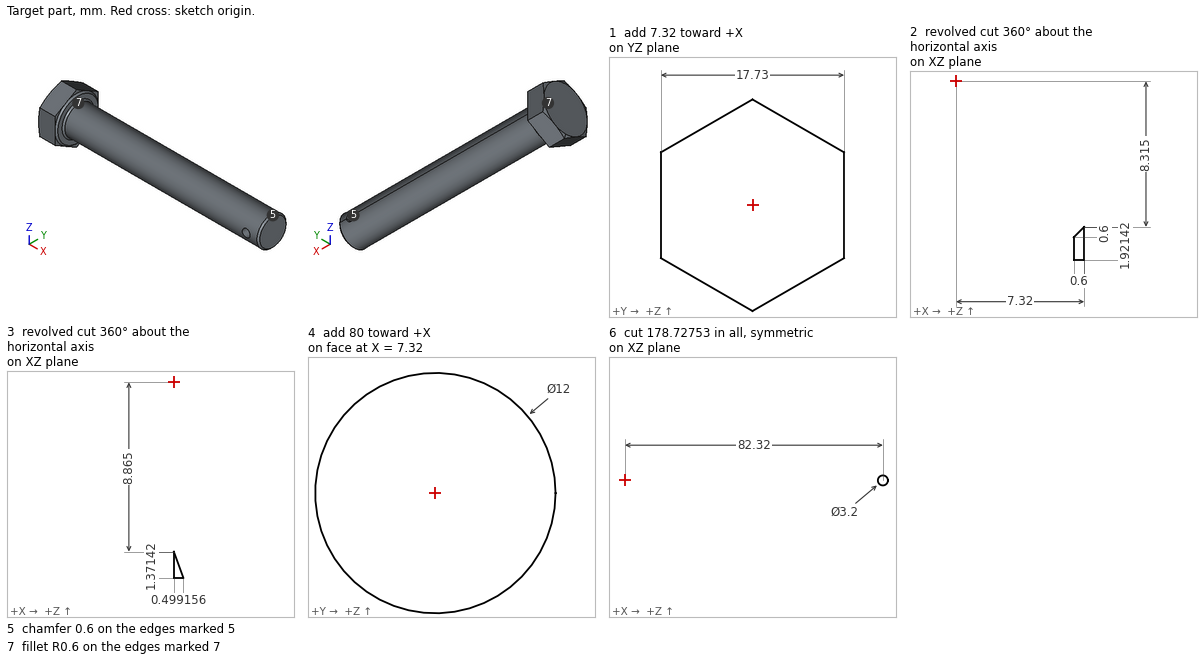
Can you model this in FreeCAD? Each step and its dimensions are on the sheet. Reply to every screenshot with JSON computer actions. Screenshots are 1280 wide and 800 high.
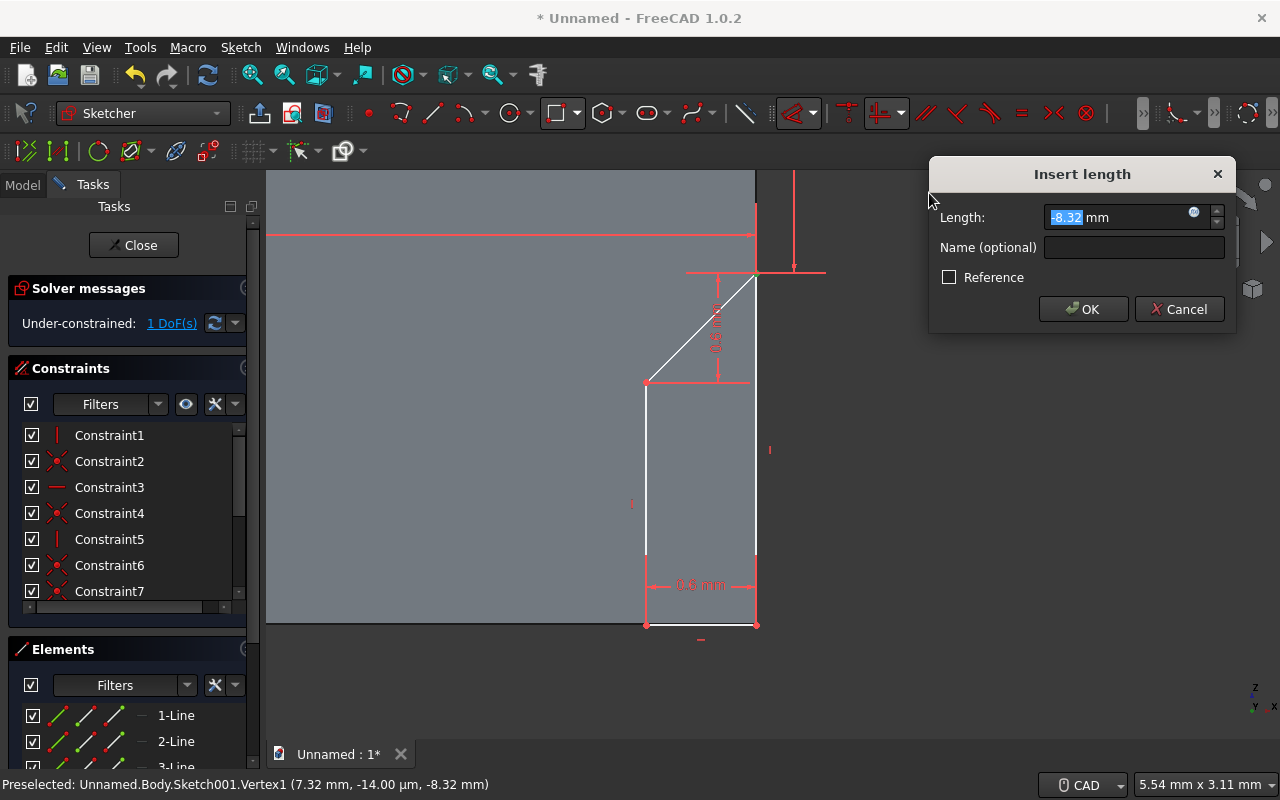
{"action": "type", "text": "-8.315"}
{"action": "key", "text": "Return"}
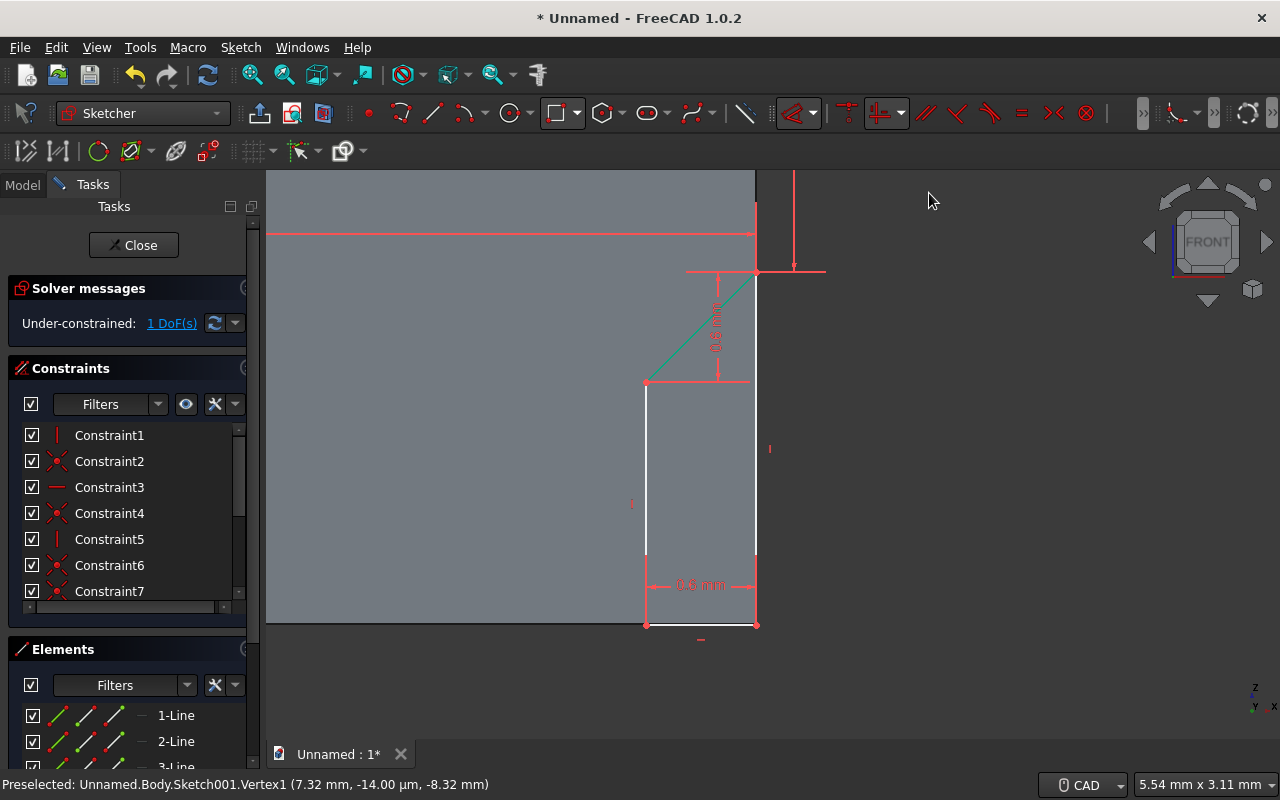
{"action": "left_click", "coordinate": [756, 378]}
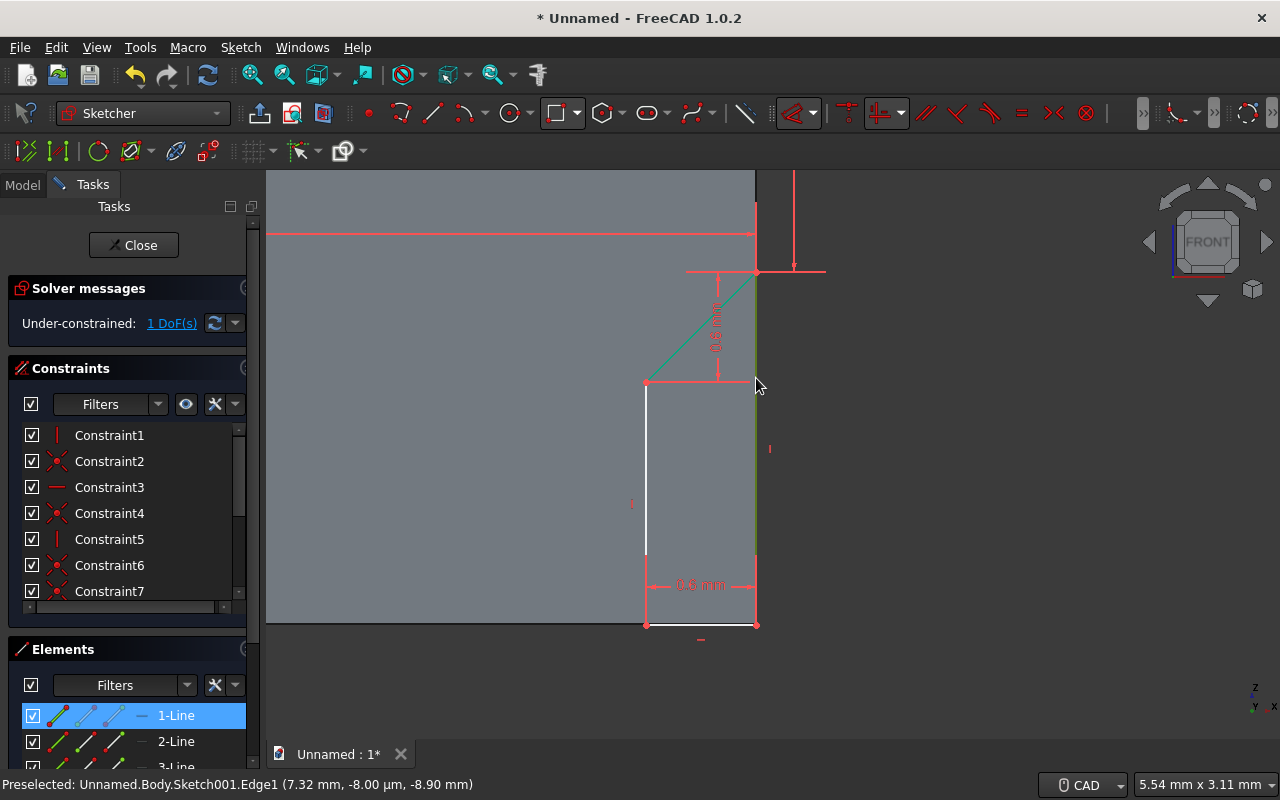
{"action": "left_click", "coordinate": [816, 114]}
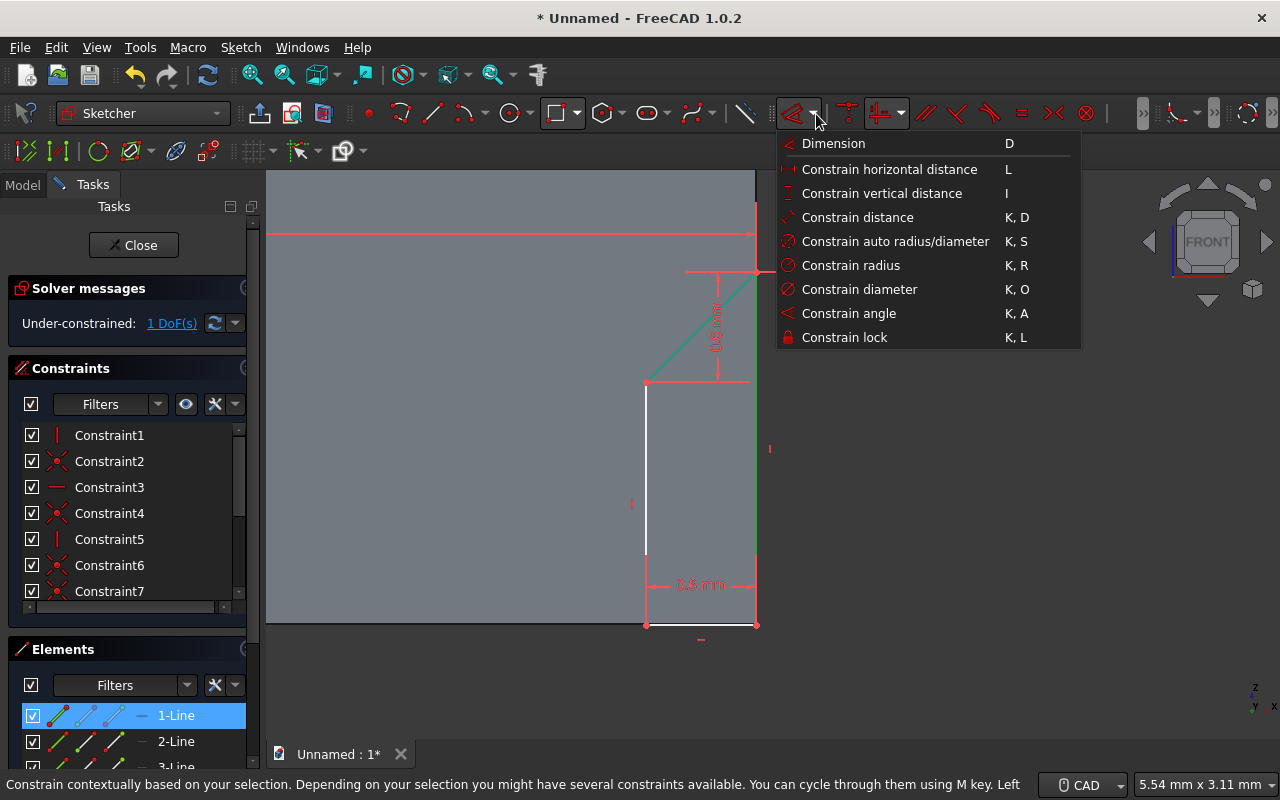
{"action": "left_click", "coordinate": [929, 193]}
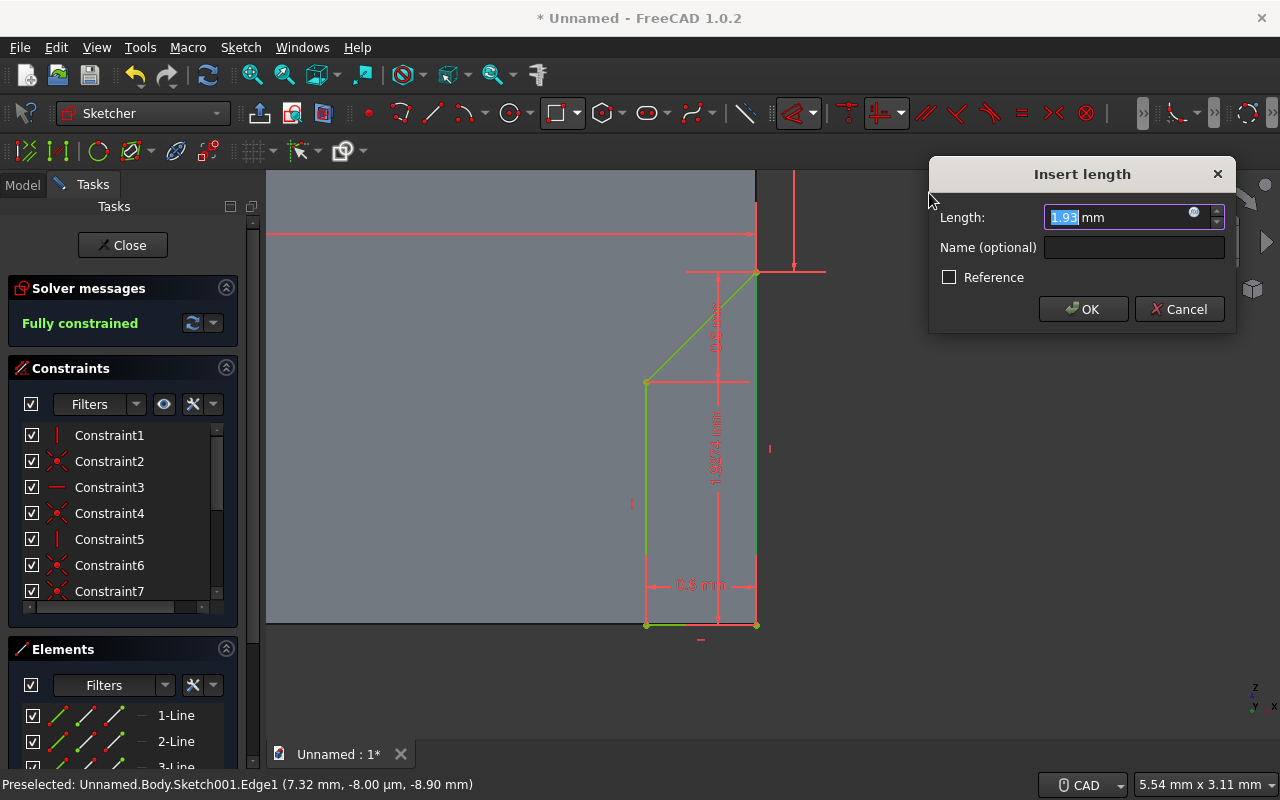
{"action": "type", "text": "1.92142"}
{"action": "key", "text": "Return"}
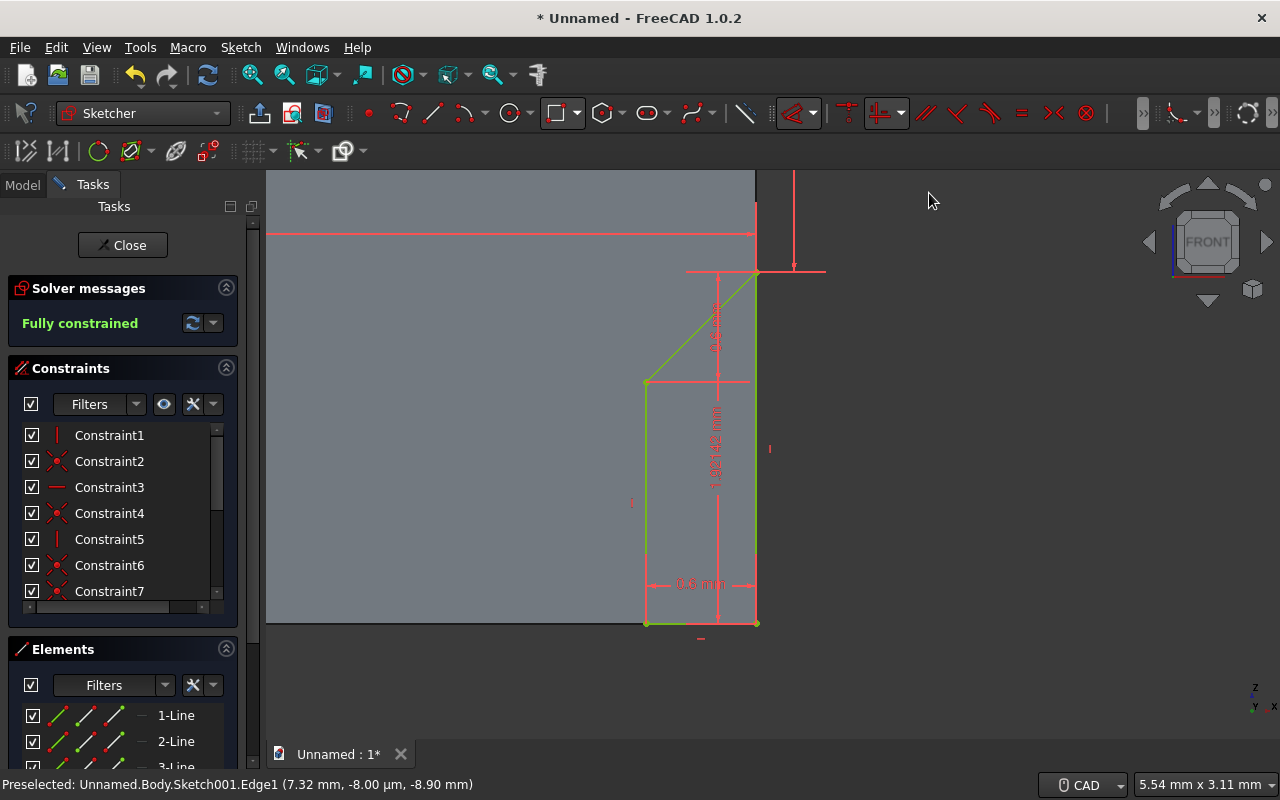
{"action": "left_click", "coordinate": [123, 245]}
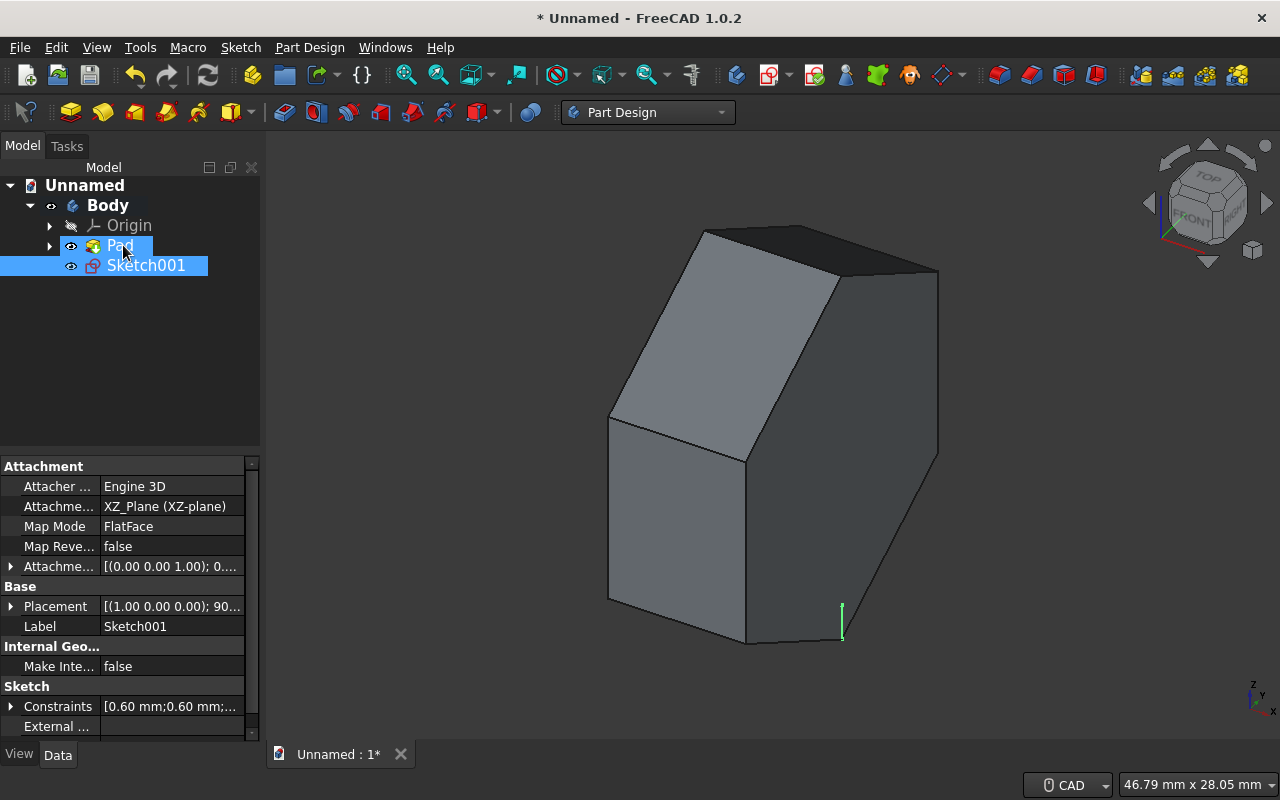
{"action": "left_click", "coordinate": [350, 112]}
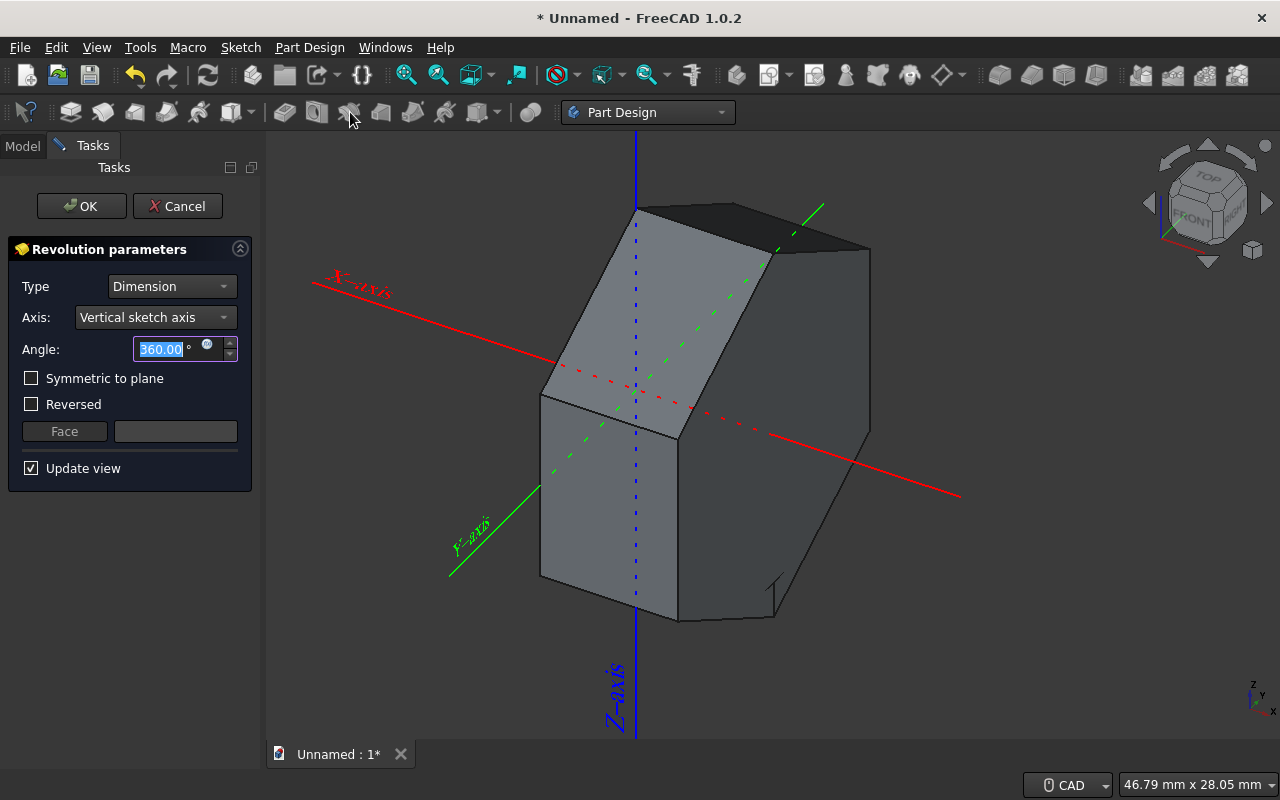
{"action": "left_click", "coordinate": [156, 318]}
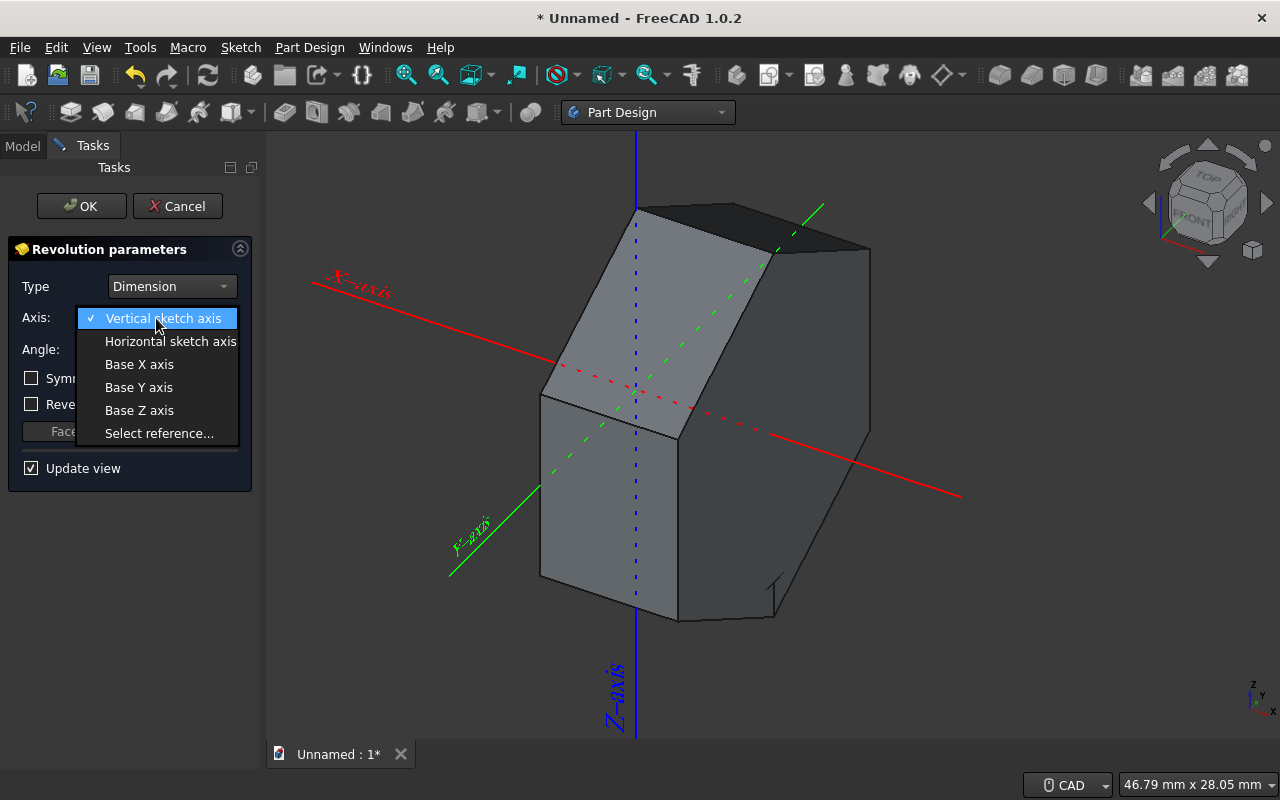
{"action": "left_click", "coordinate": [156, 342]}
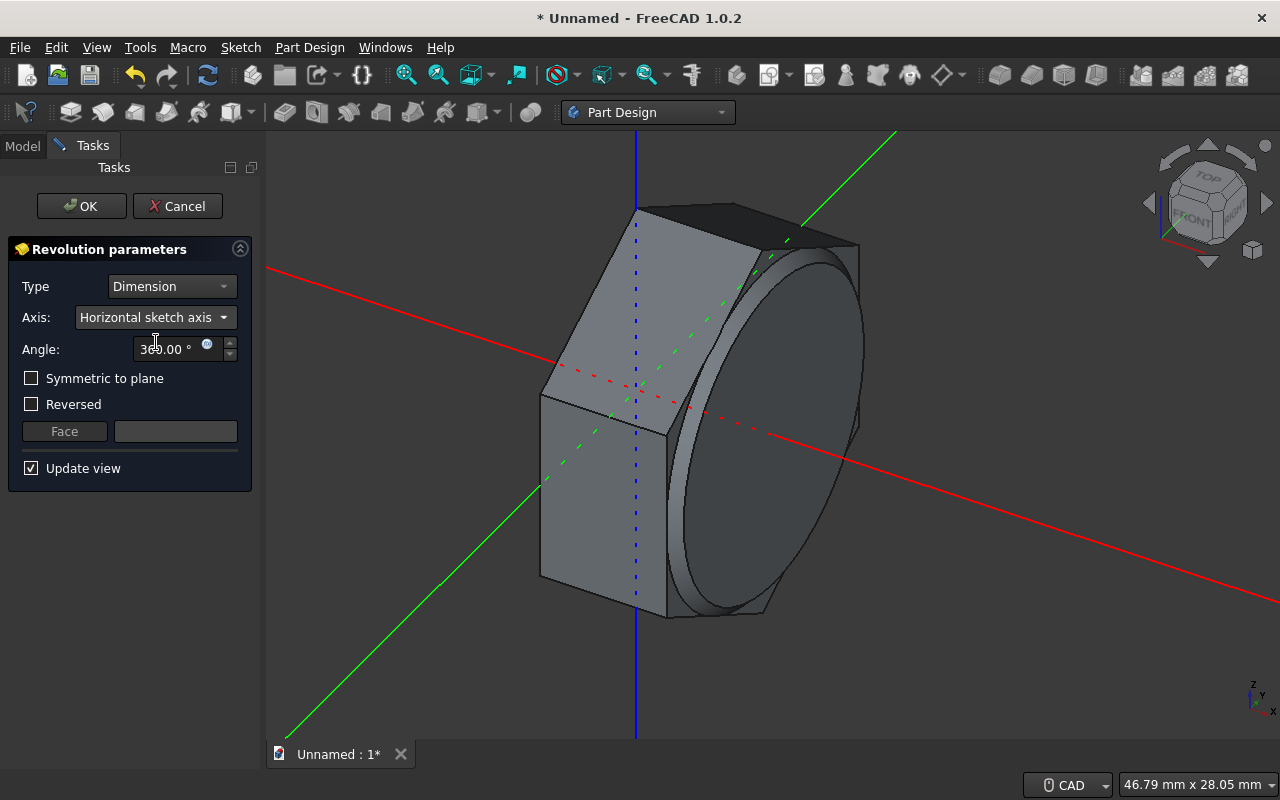
{"action": "left_click", "coordinate": [82, 206]}